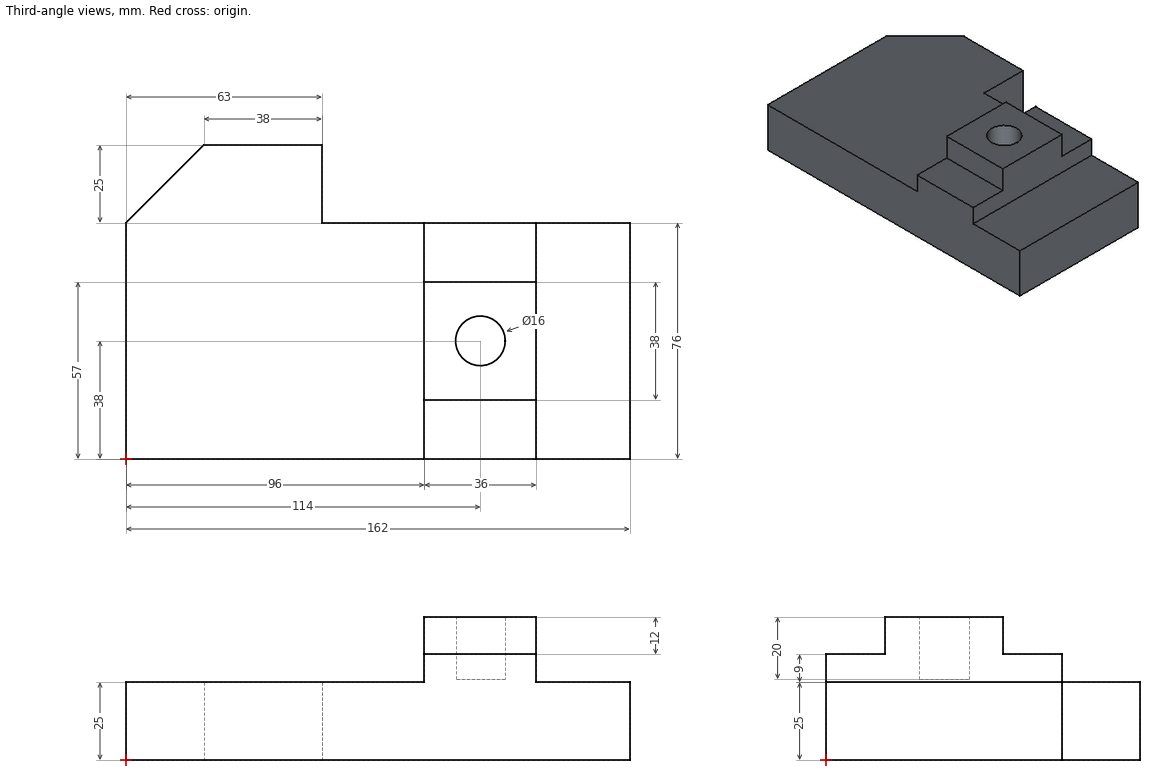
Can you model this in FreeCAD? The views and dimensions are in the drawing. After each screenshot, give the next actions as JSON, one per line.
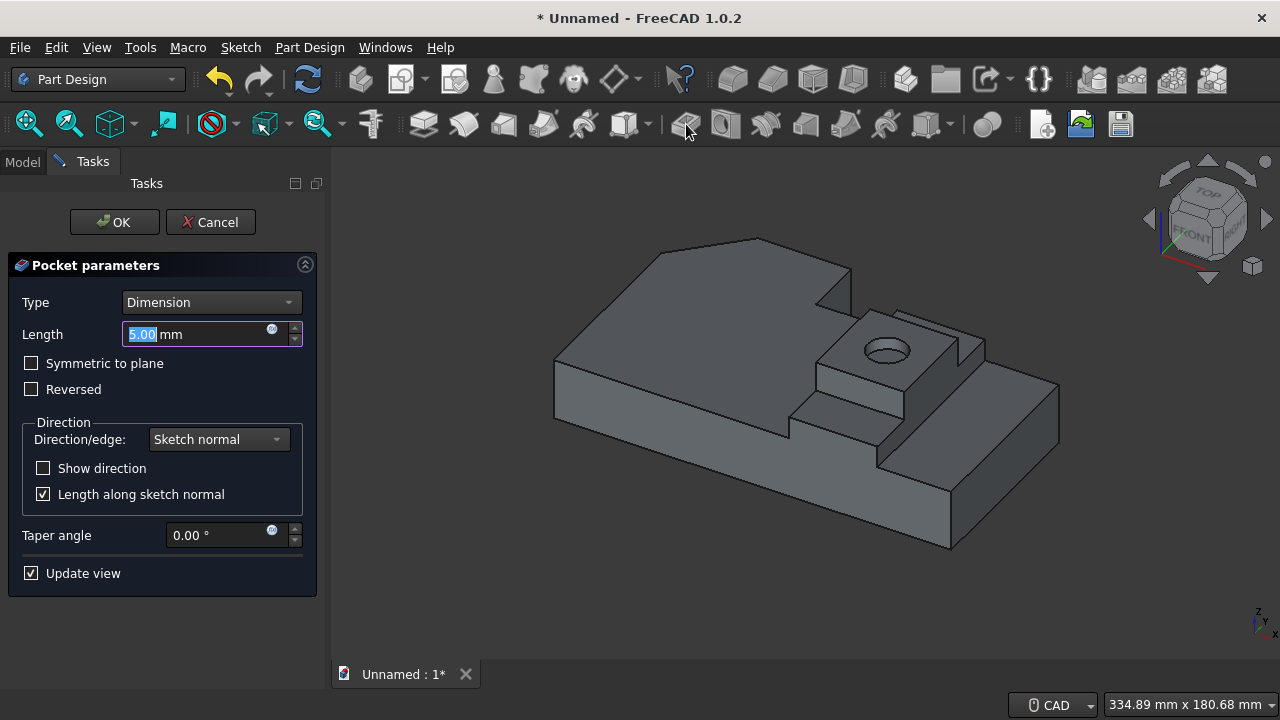
{"action": "type", "text": "20"}
{"action": "key", "text": "Tab"}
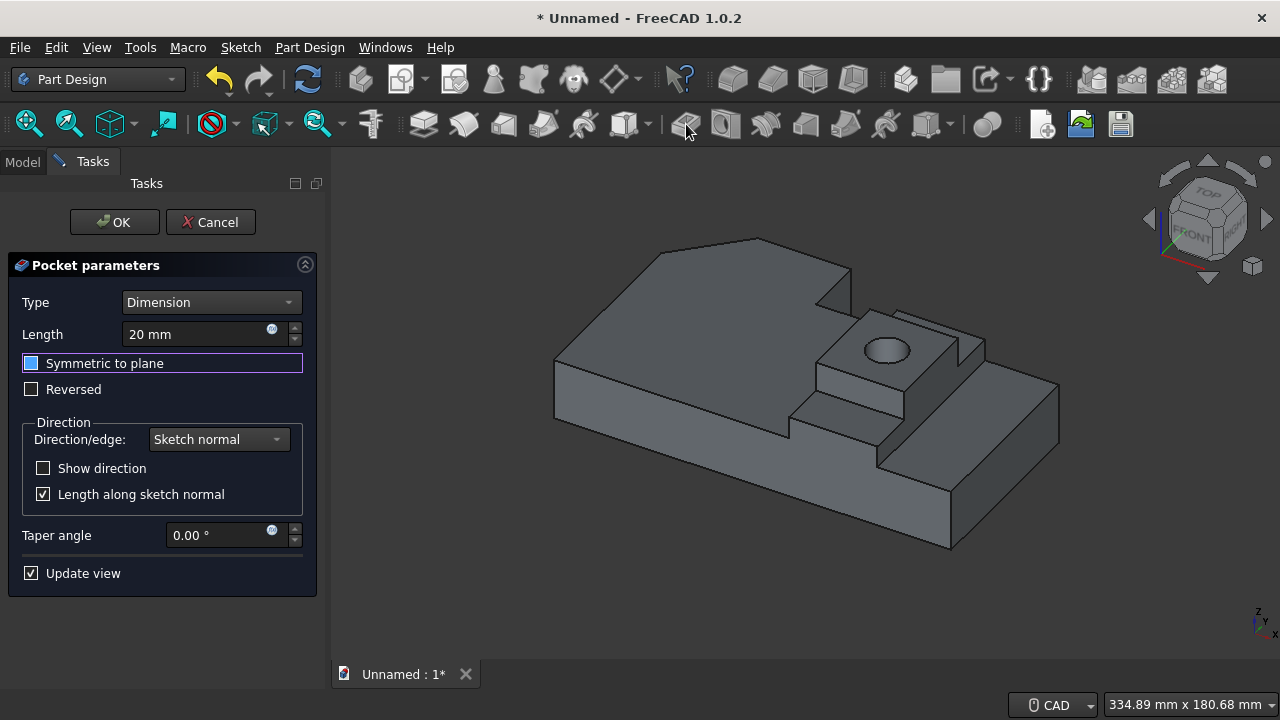
{"action": "left_click", "coordinate": [115, 222]}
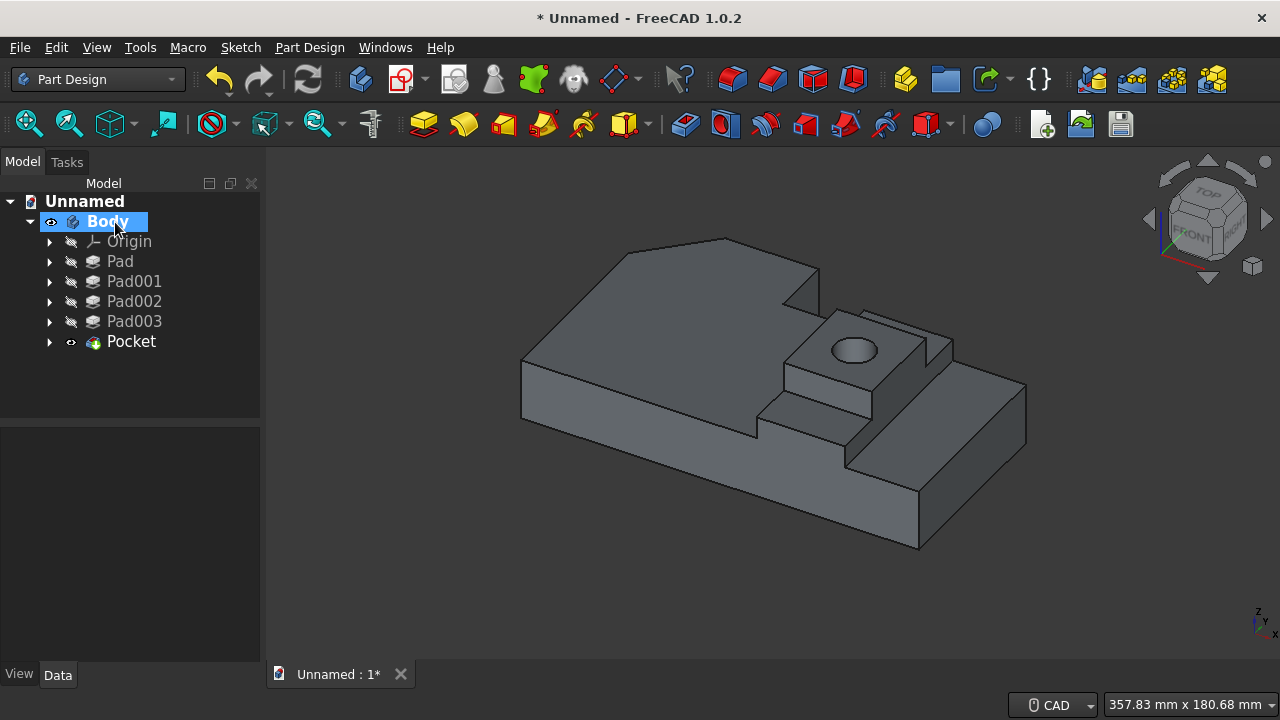
{"action": "key", "text": "0"}